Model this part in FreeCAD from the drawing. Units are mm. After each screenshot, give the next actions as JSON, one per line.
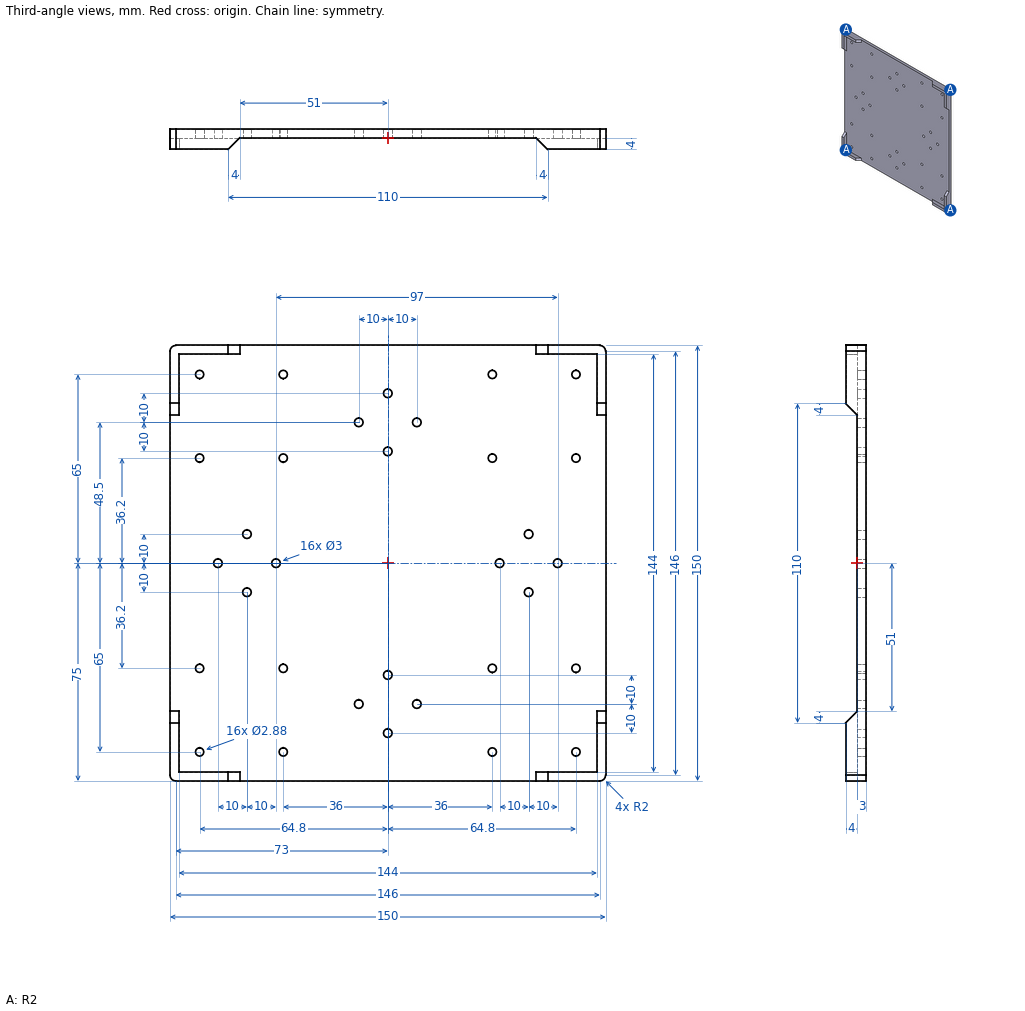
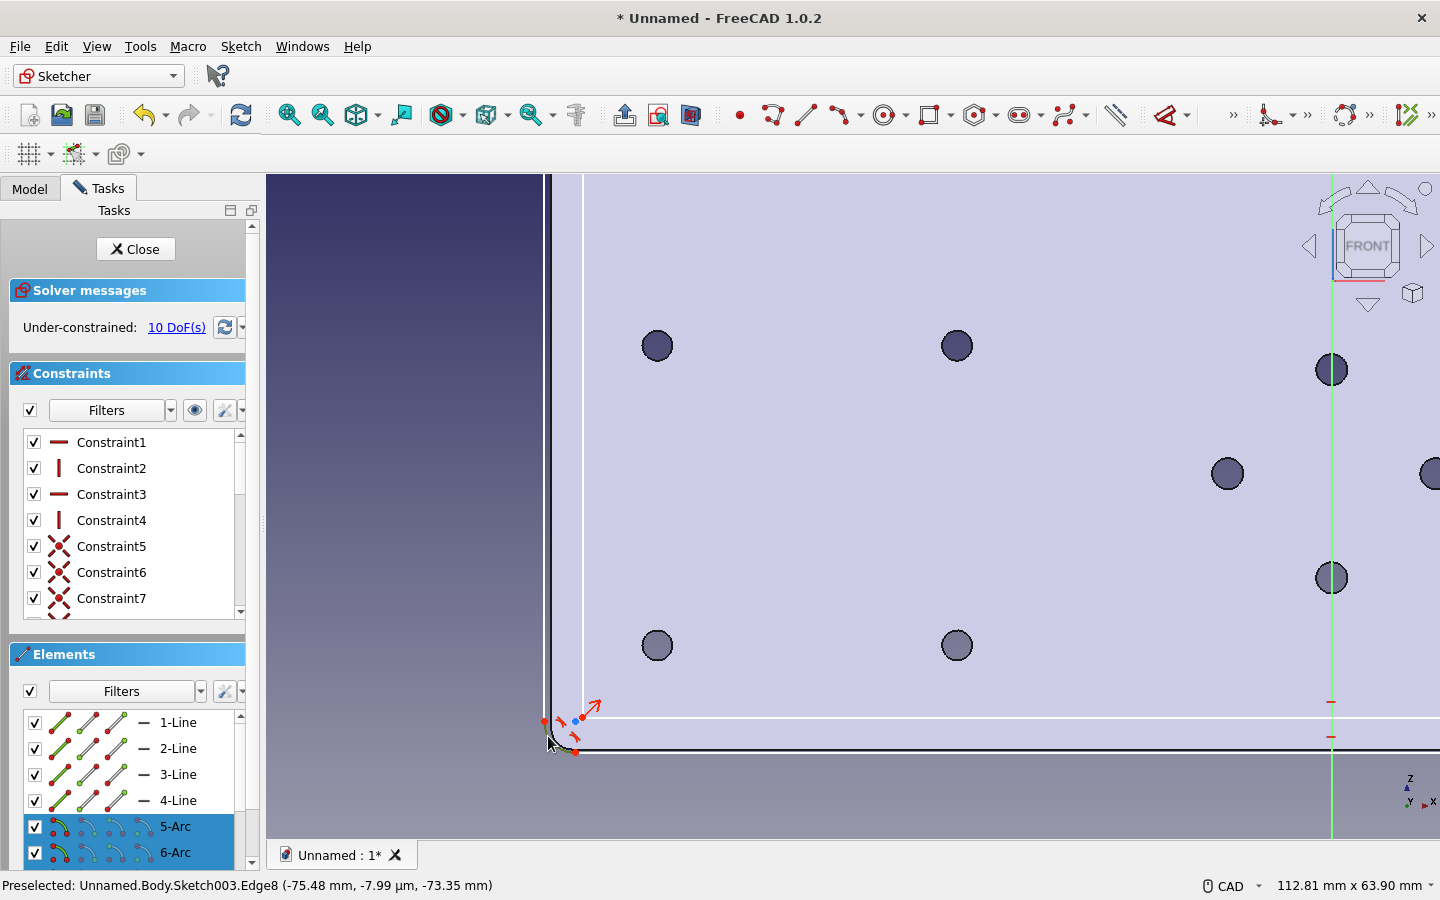
{"action": "key", "text": "e"}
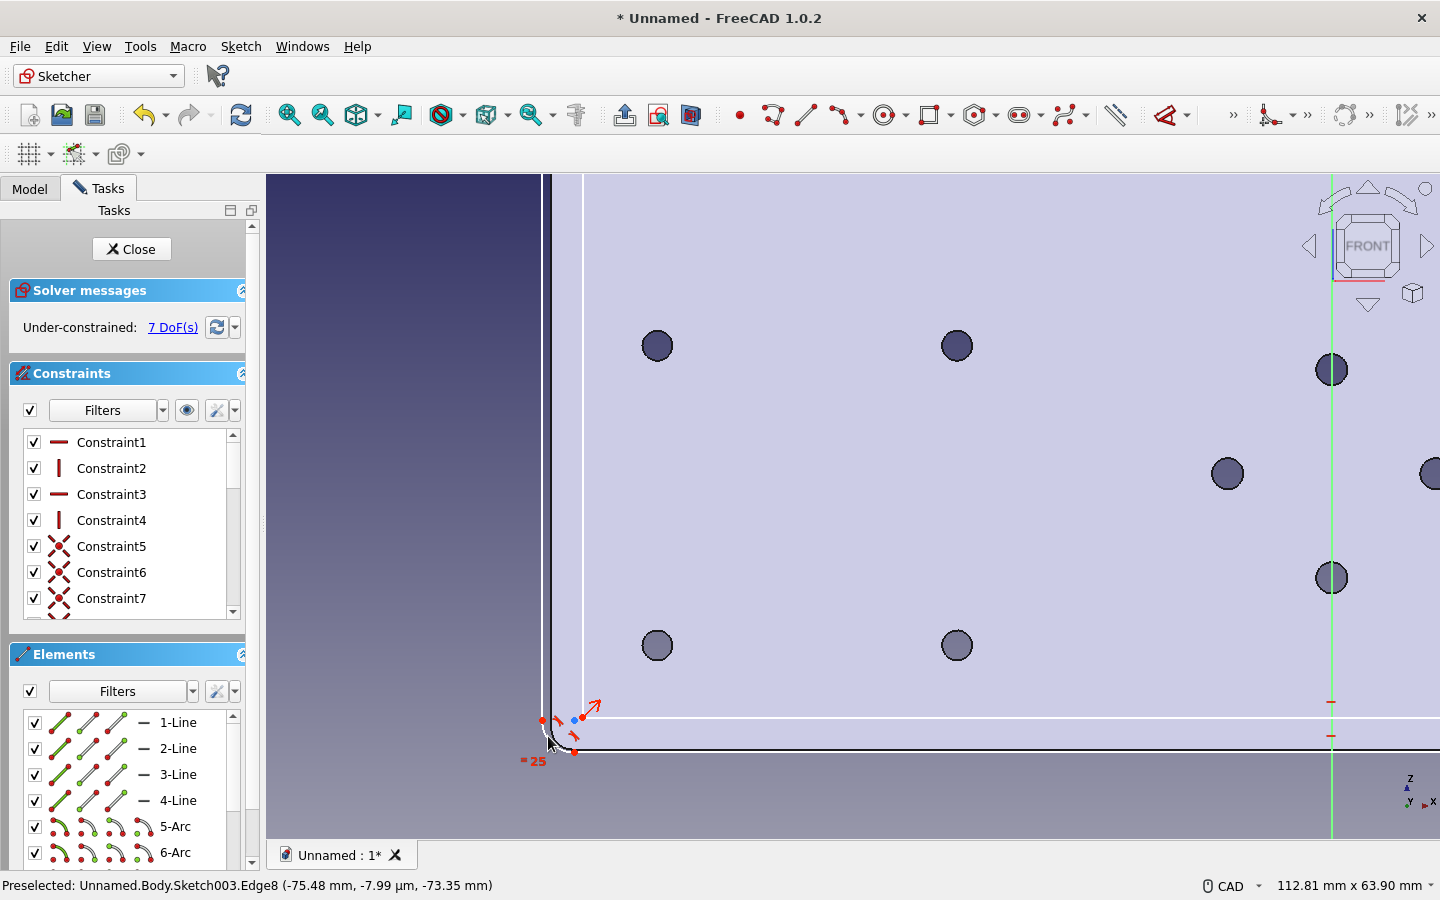
{"action": "left_click", "coordinate": [1164, 116]}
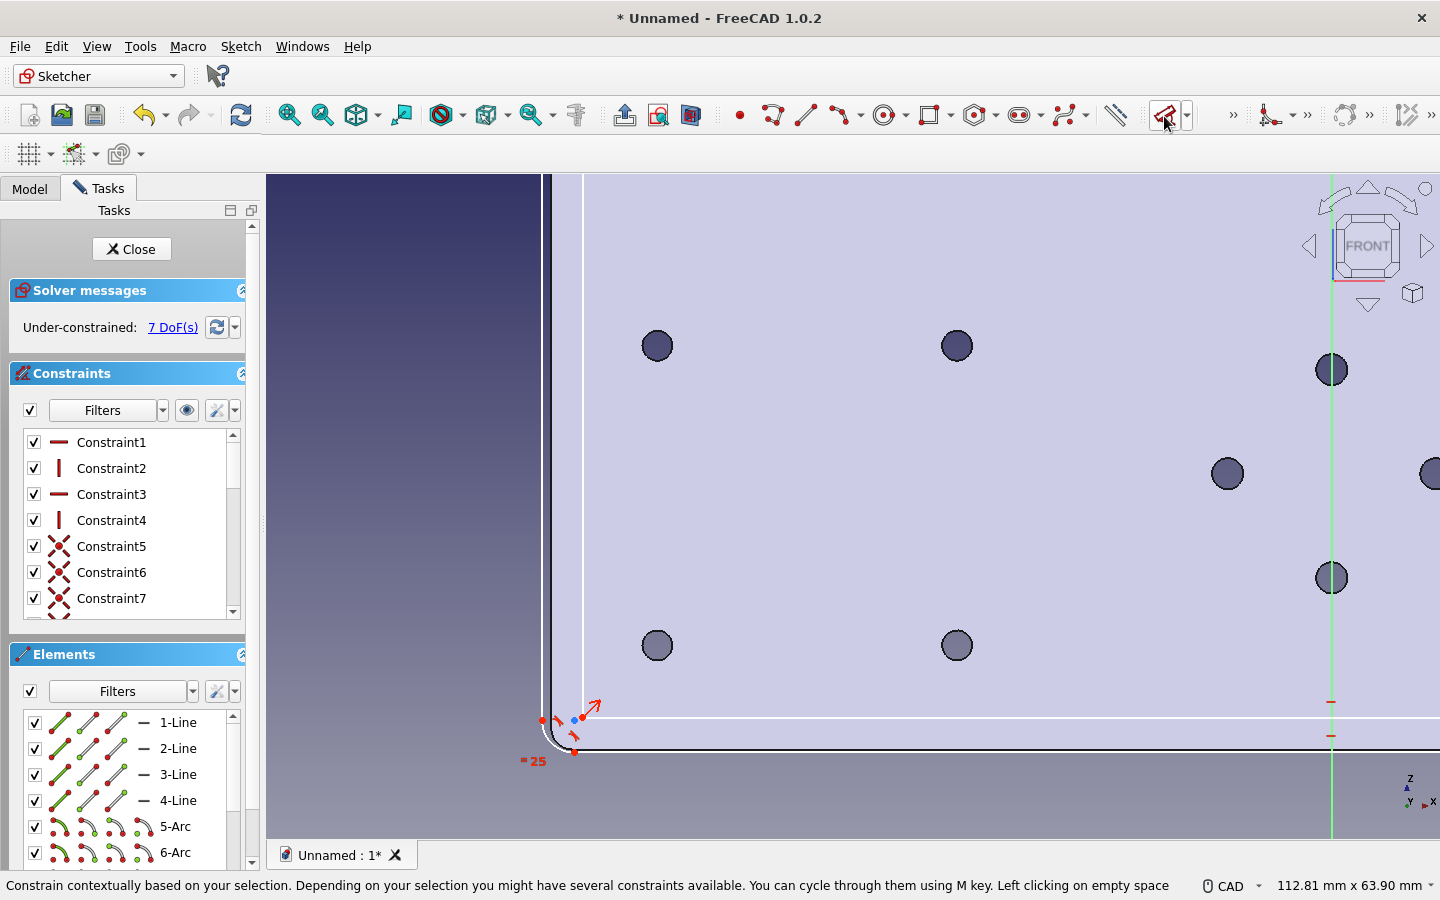
{"action": "scroll", "coordinate": [549, 738], "scroll_direction": "down", "scroll_amount": 6}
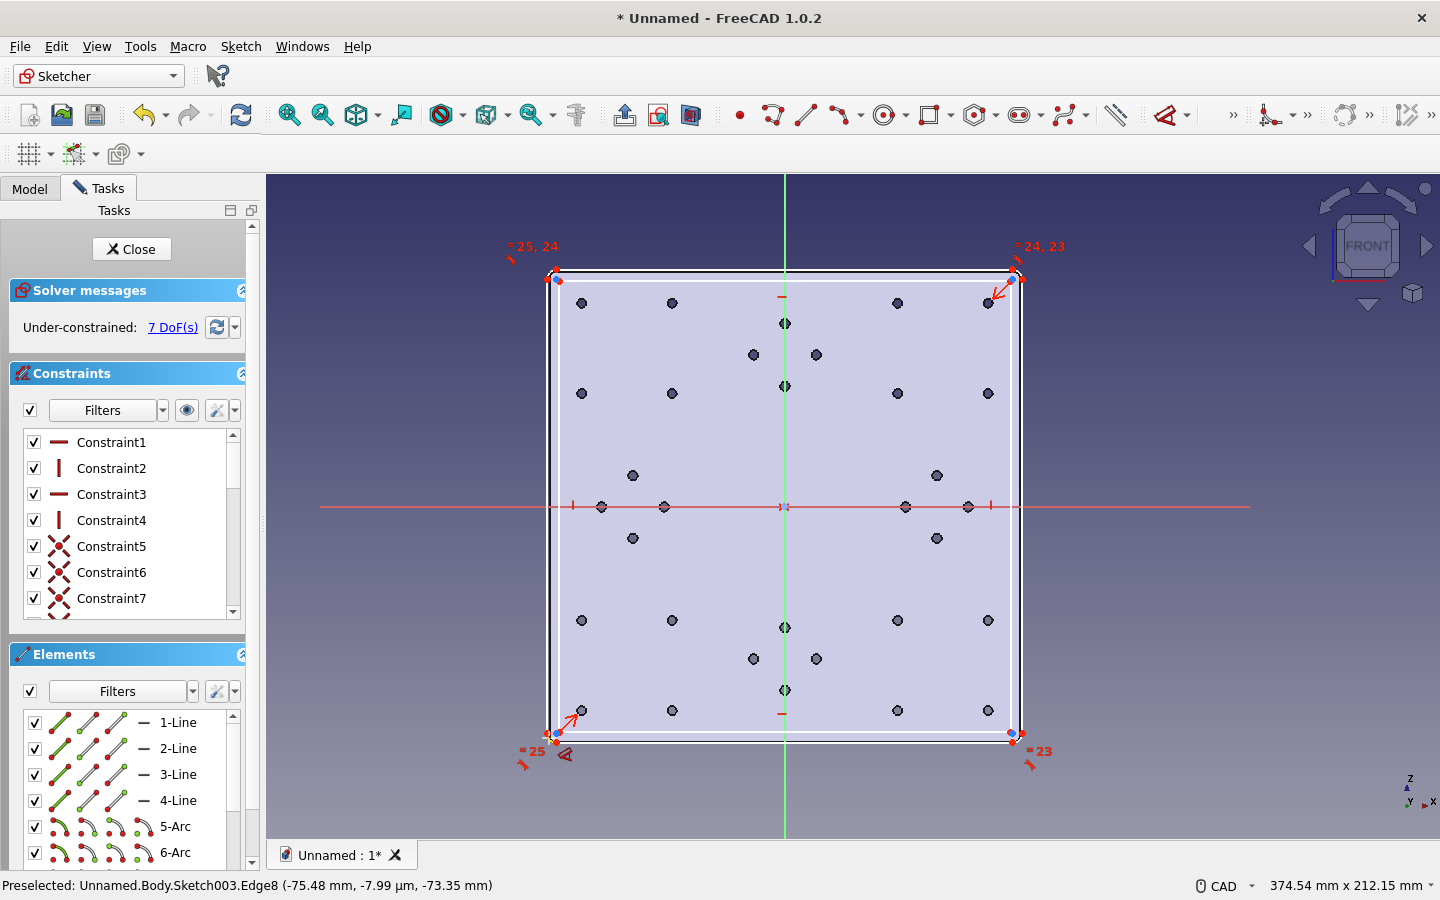
{"action": "scroll", "coordinate": [1017, 742], "scroll_direction": "up", "scroll_amount": 10}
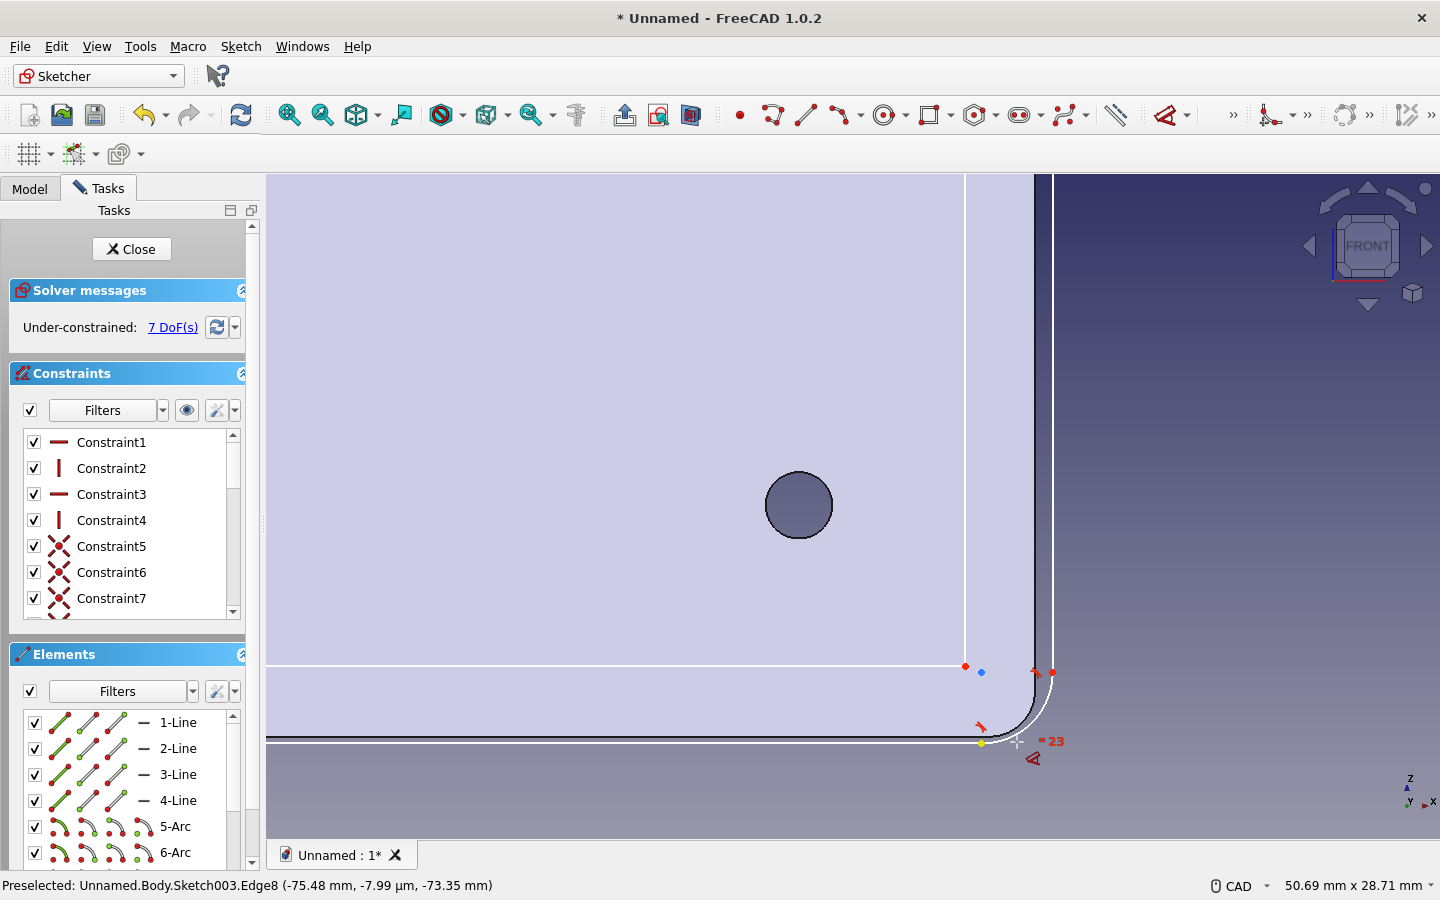
{"action": "left_click", "coordinate": [1014, 736]}
{"action": "left_click", "coordinate": [1029, 765]}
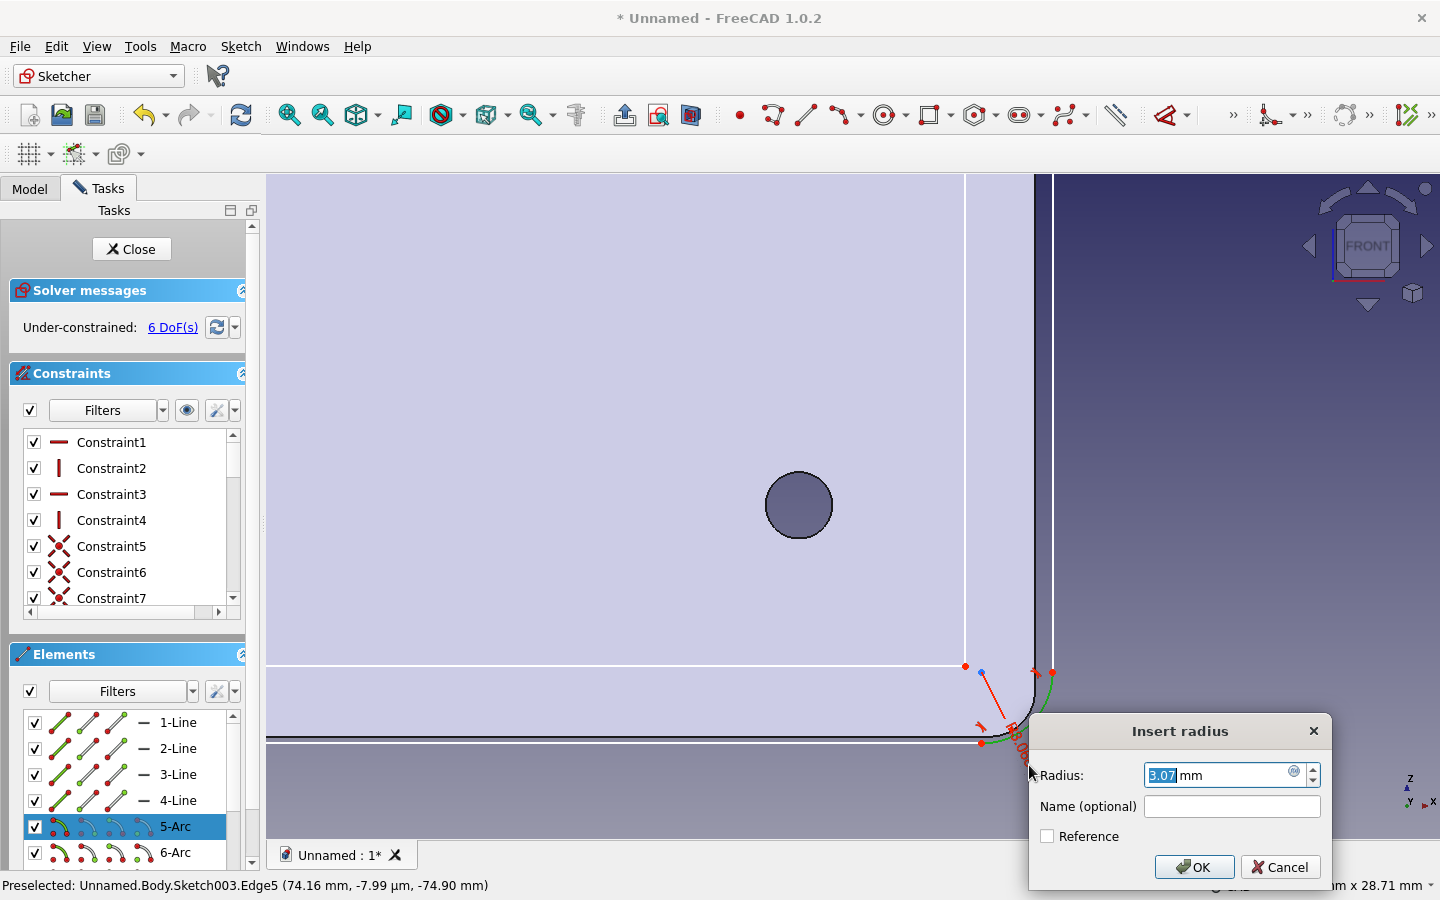
{"action": "type", "text": "2"}
{"action": "key", "text": "Return"}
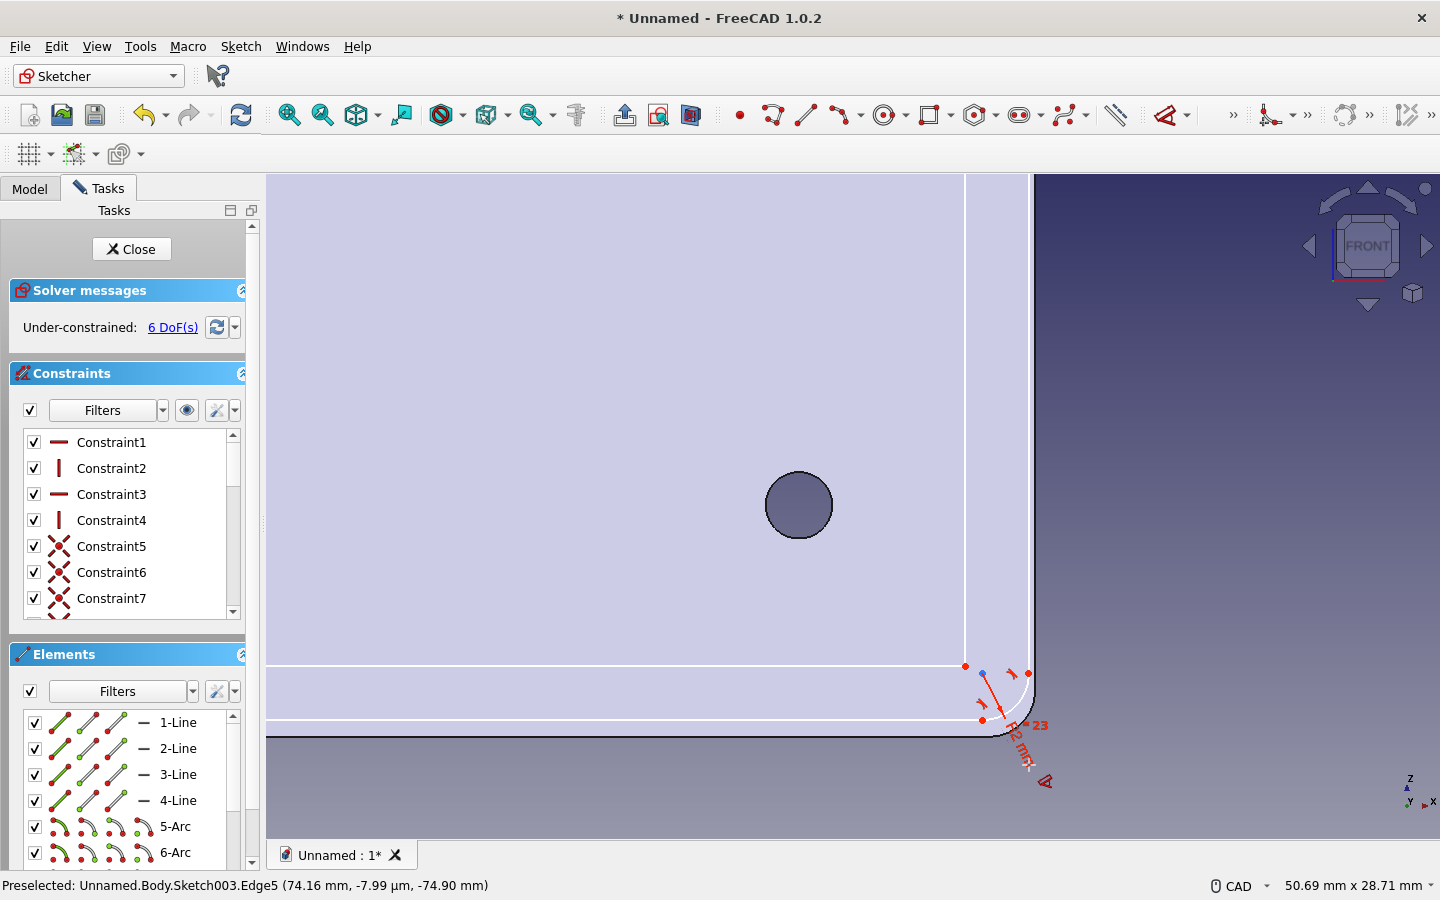
{"action": "scroll", "coordinate": [1017, 742], "scroll_direction": "down", "scroll_amount": 10}